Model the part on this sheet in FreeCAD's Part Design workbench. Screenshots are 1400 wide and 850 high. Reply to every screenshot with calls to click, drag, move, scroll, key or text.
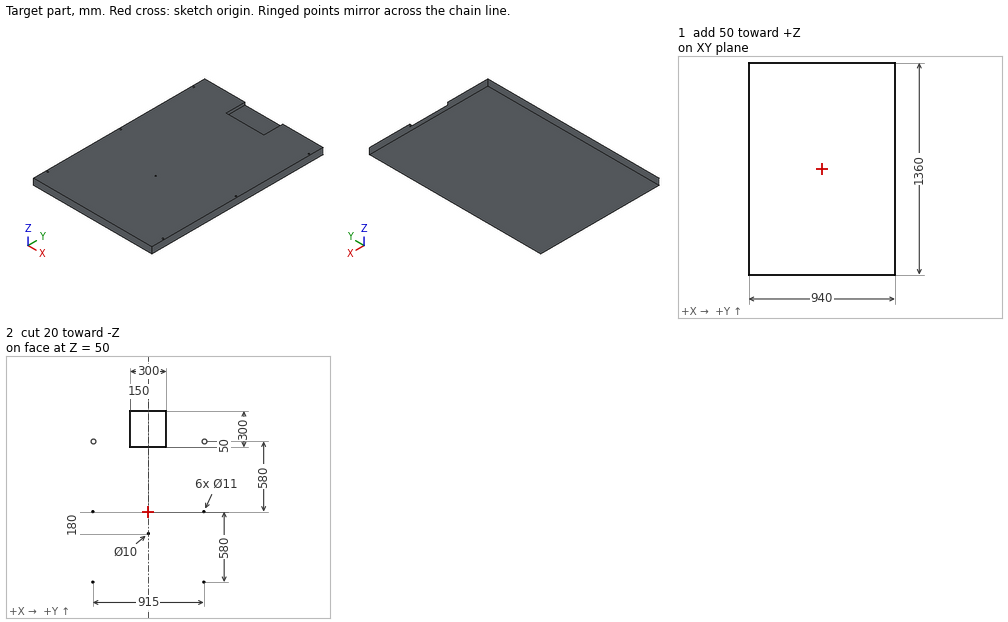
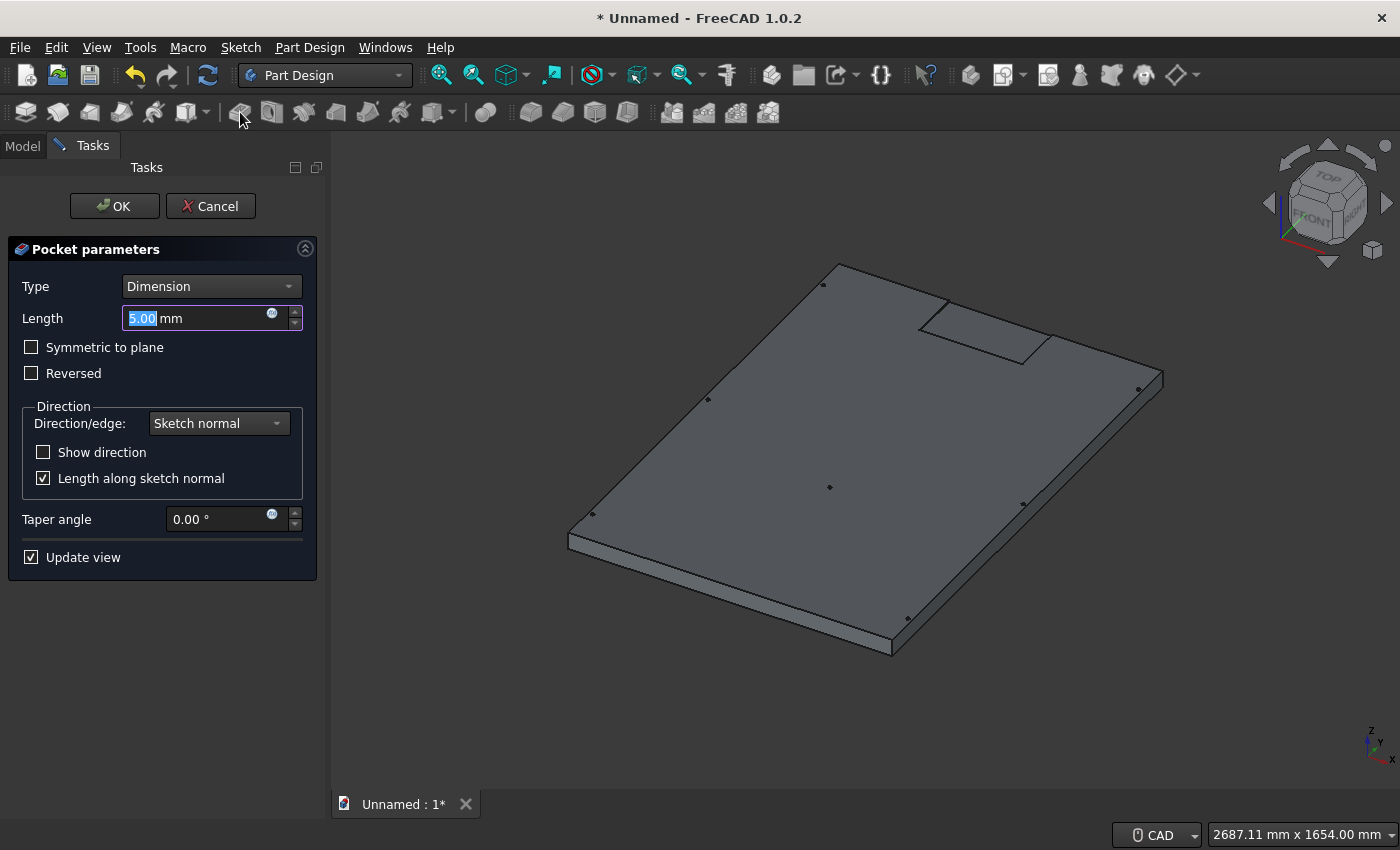
text(20)
key(Tab)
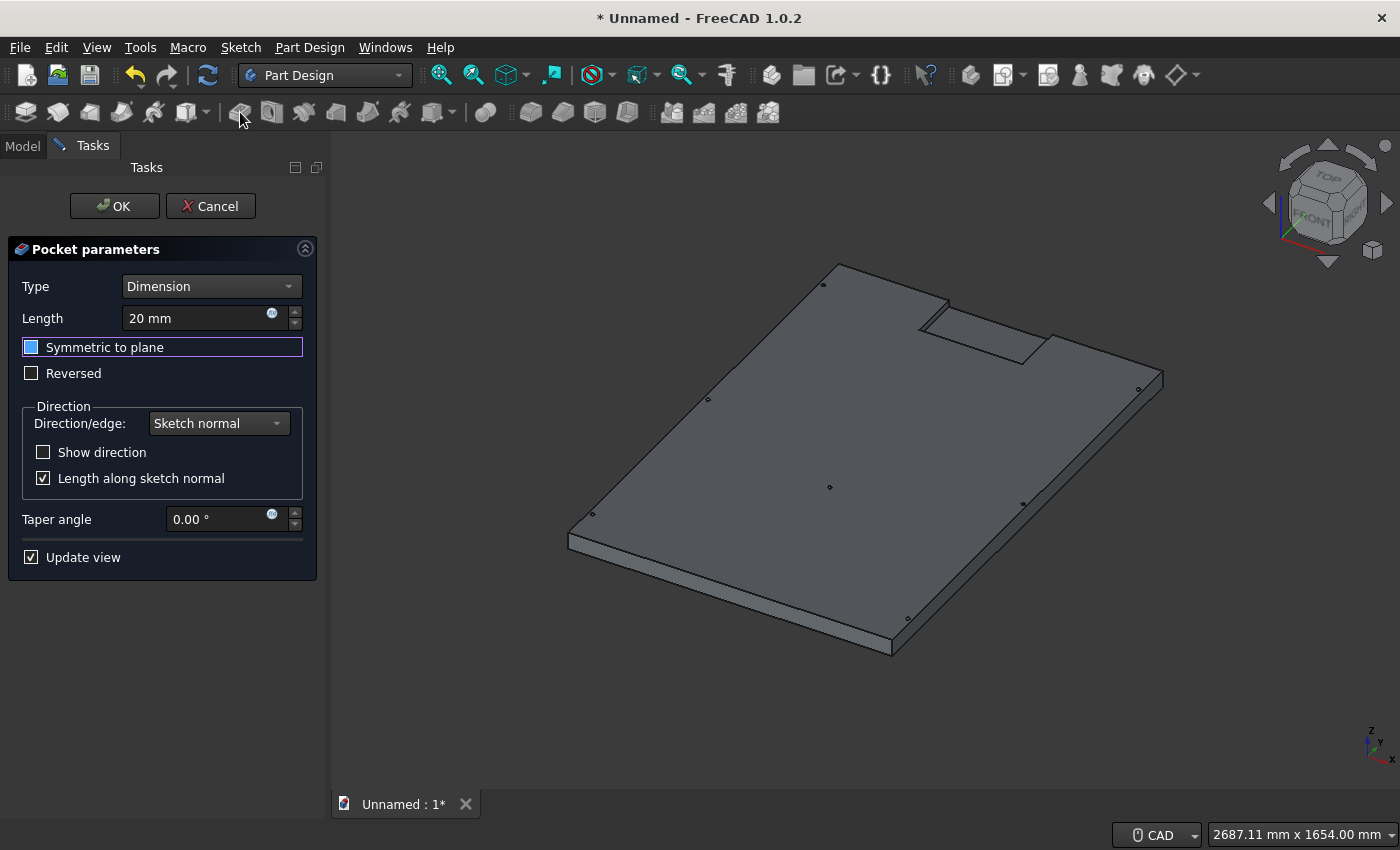
click(115, 206)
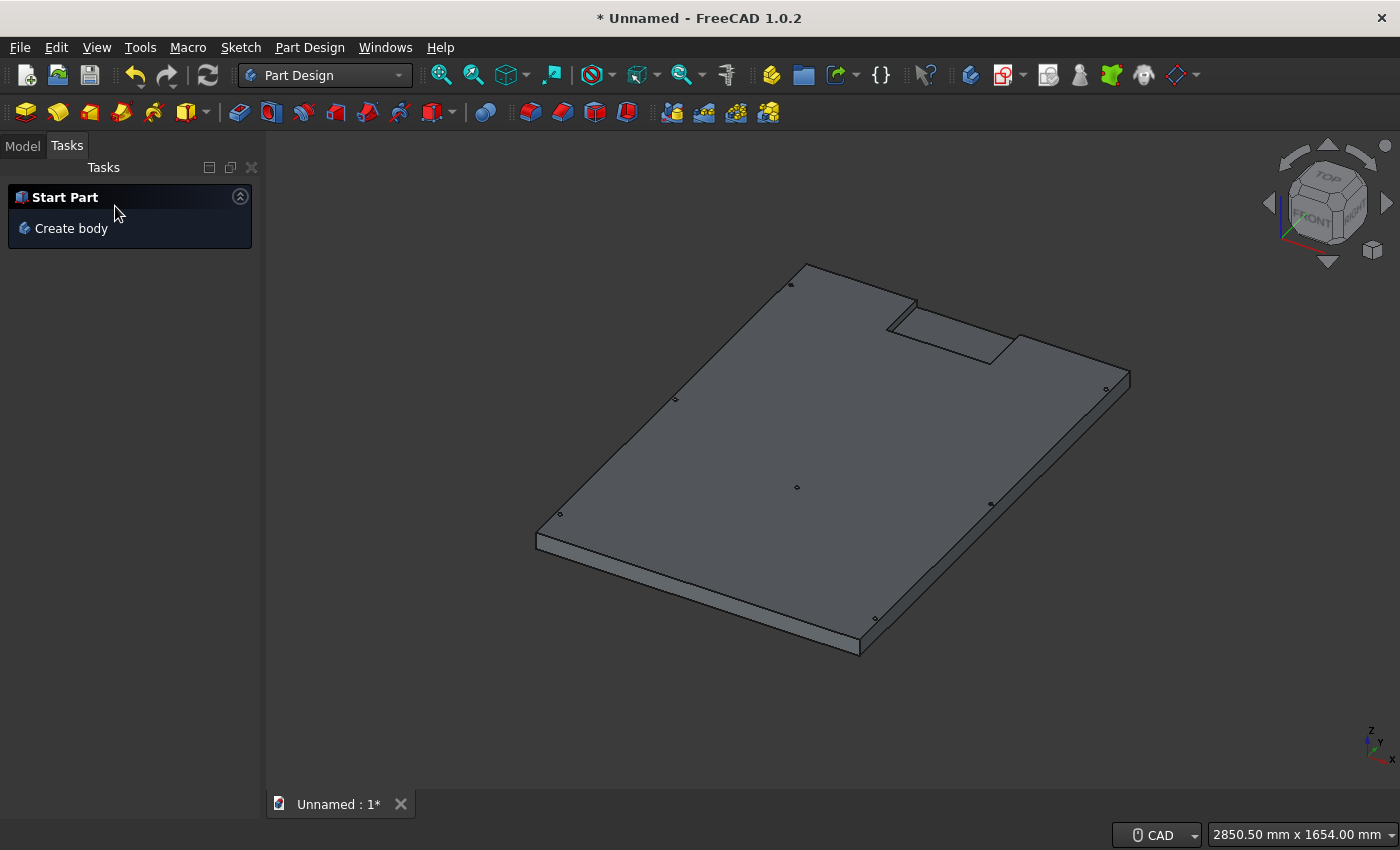
key(0)